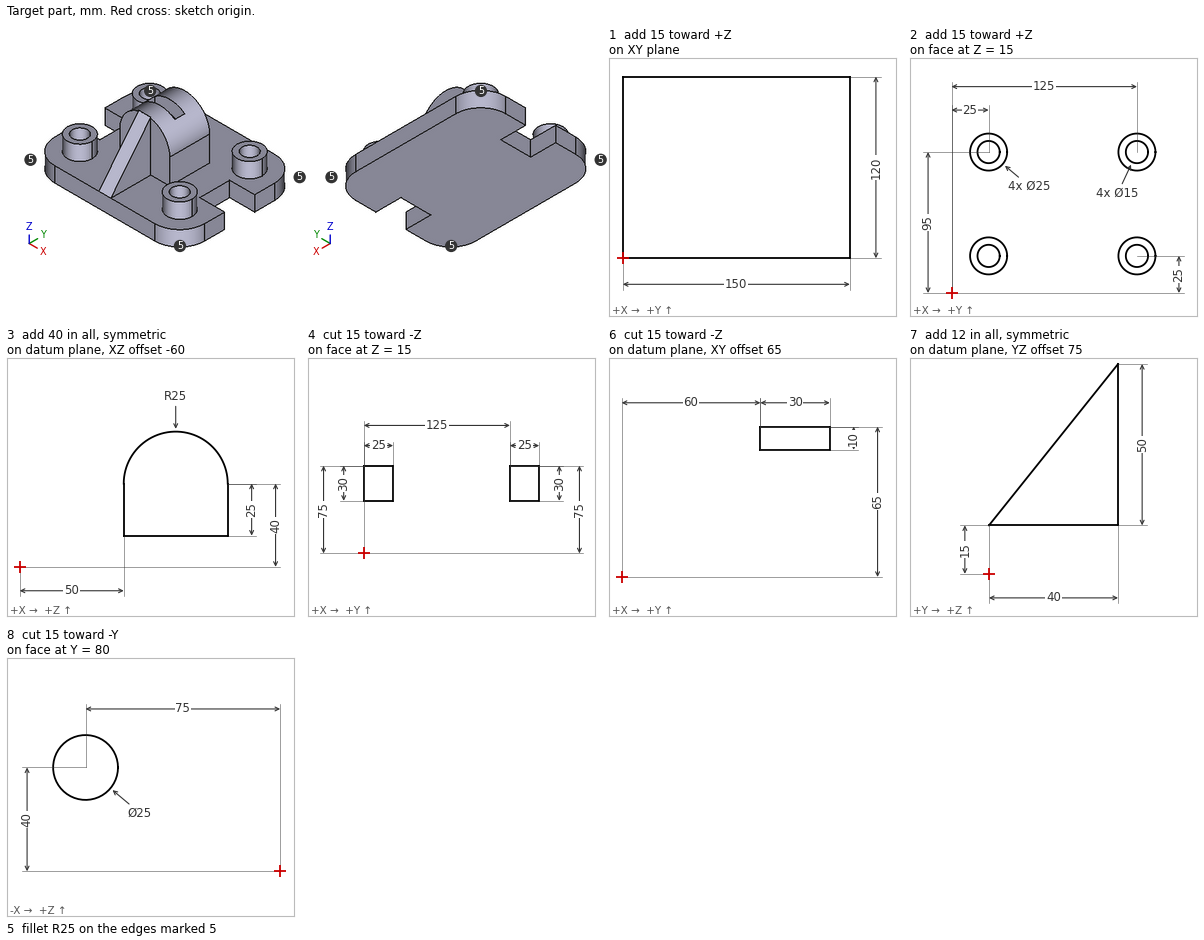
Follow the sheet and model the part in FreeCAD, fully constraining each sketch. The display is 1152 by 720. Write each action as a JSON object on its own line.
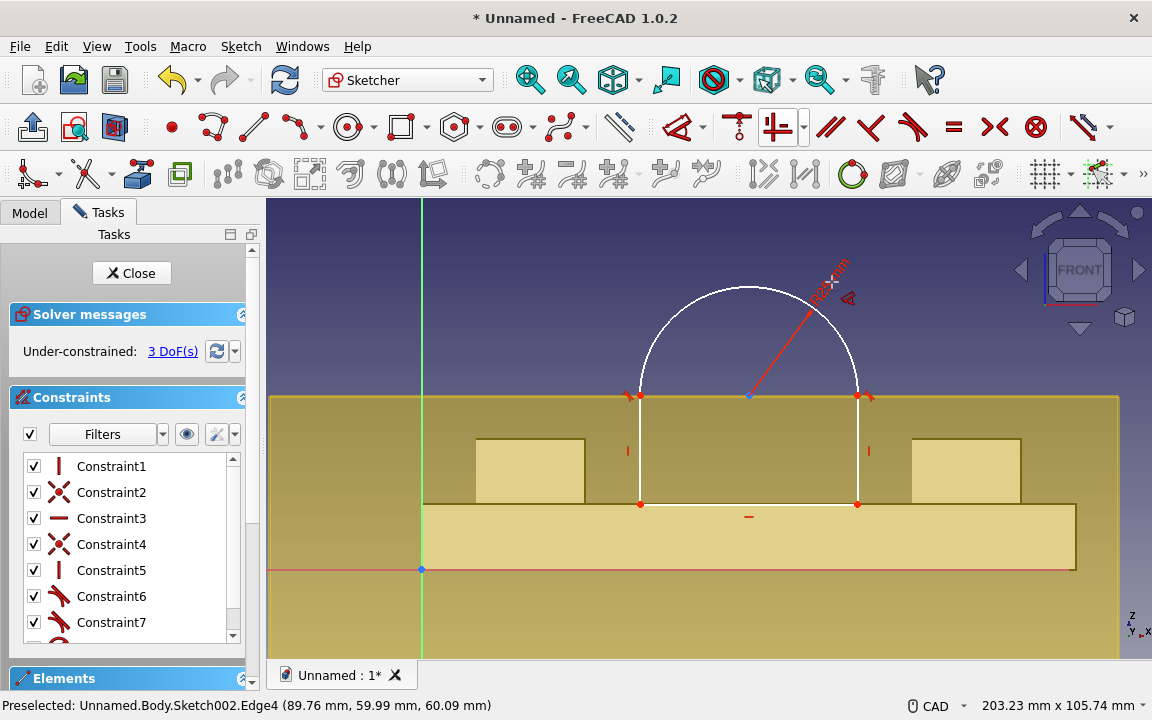
{"action": "left_click", "coordinate": [858, 429]}
{"action": "left_click", "coordinate": [892, 450]}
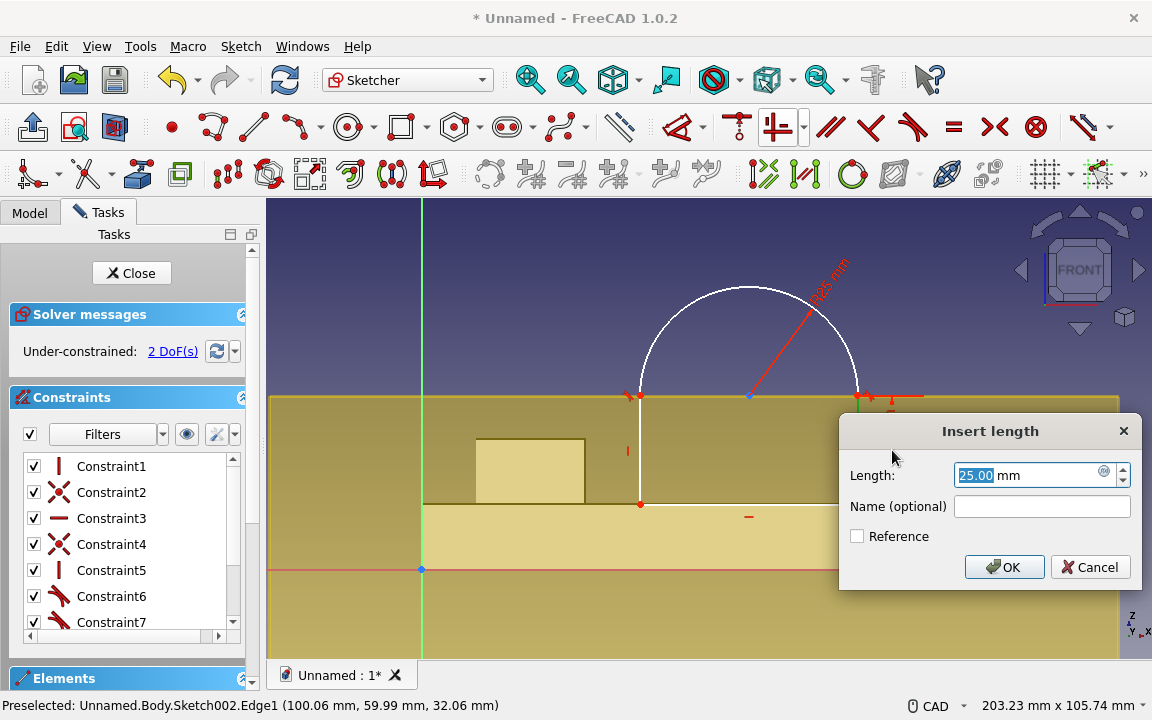
{"action": "type", "text": "25"}
{"action": "key", "text": "Return"}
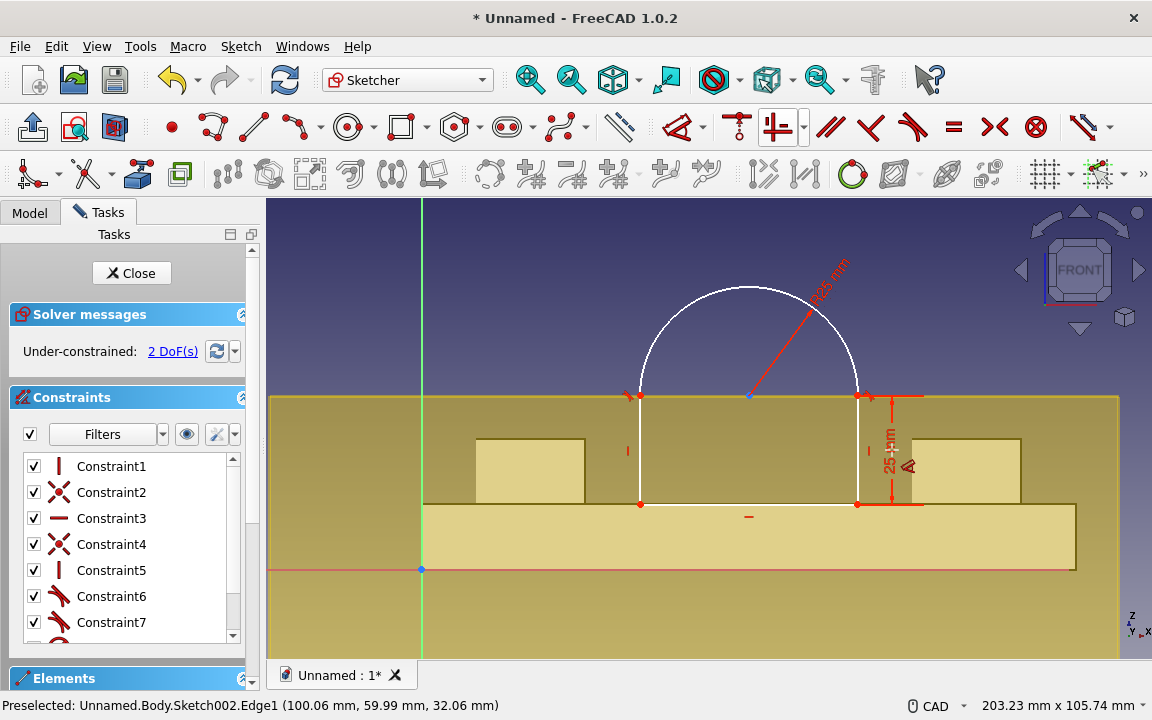
{"action": "left_click", "coordinate": [858, 396]}
{"action": "left_click", "coordinate": [892, 483]}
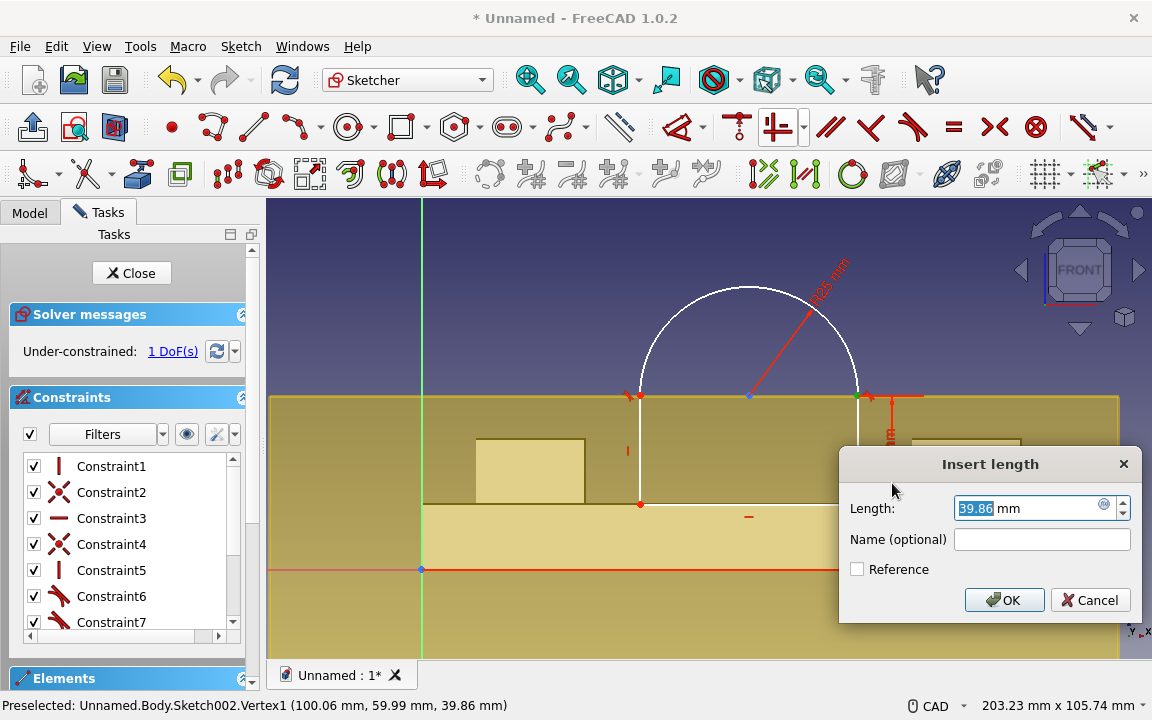
{"action": "type", "text": "40"}
{"action": "key", "text": "Return"}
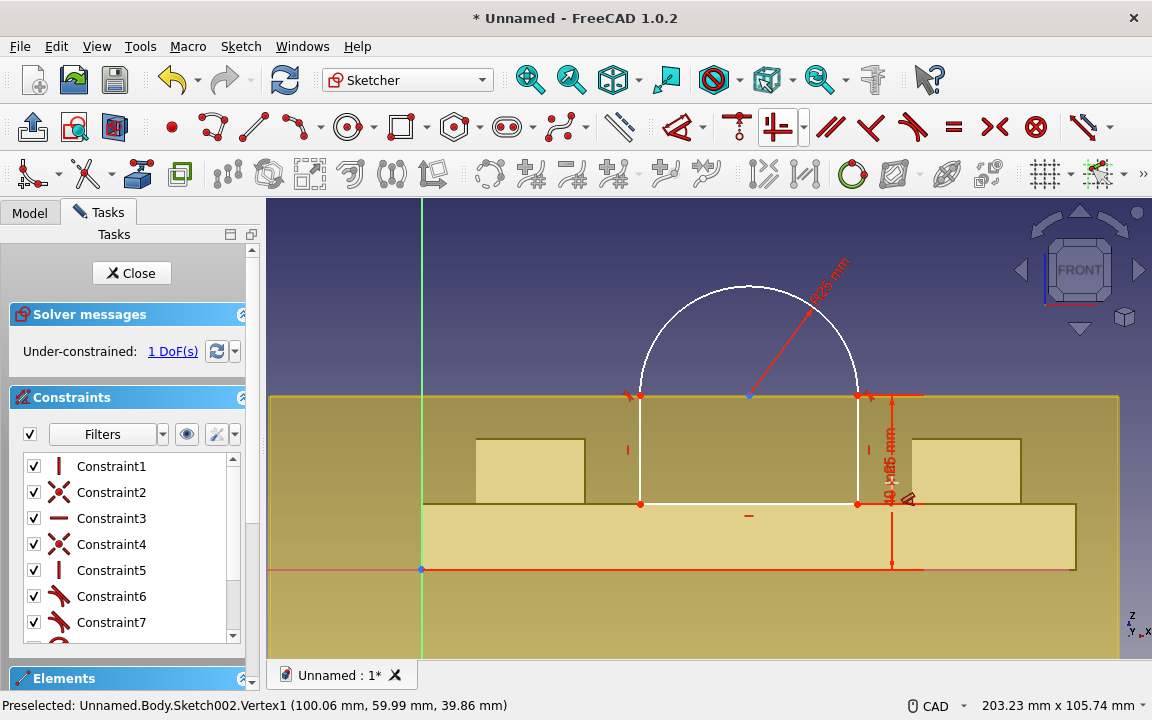
{"action": "left_click", "coordinate": [640, 504]}
{"action": "left_click", "coordinate": [531, 604]}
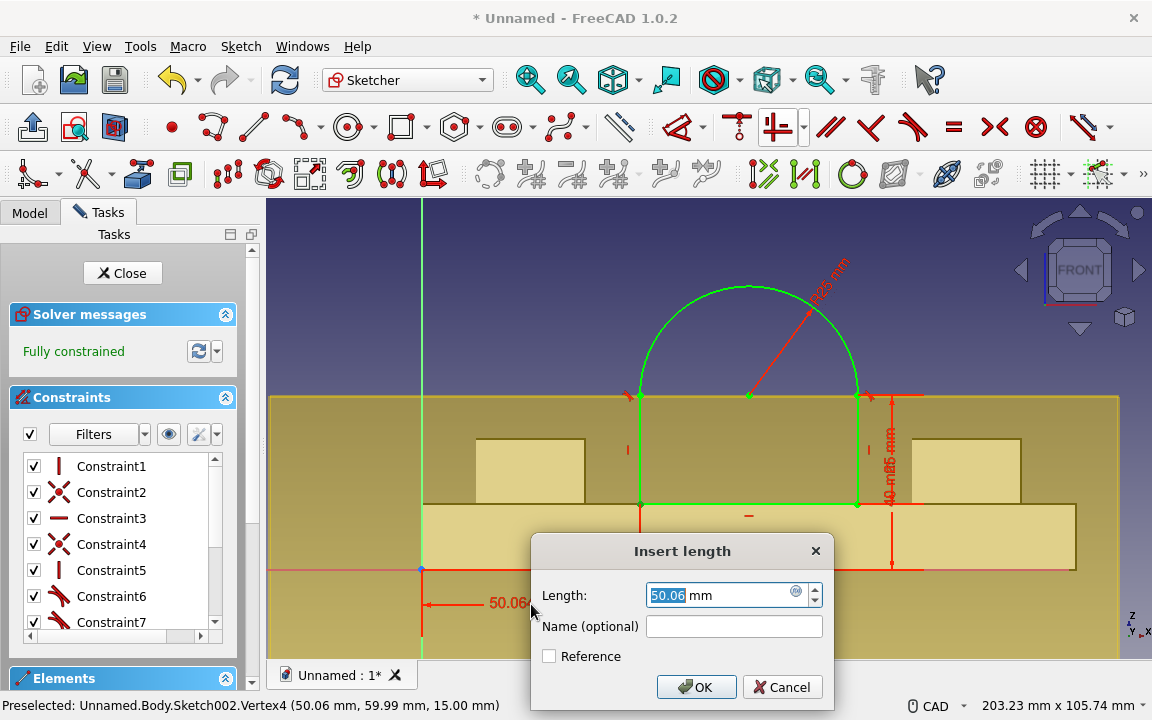
{"action": "type", "text": "50"}
{"action": "key", "text": "Return"}
{"action": "key", "text": "Escape"}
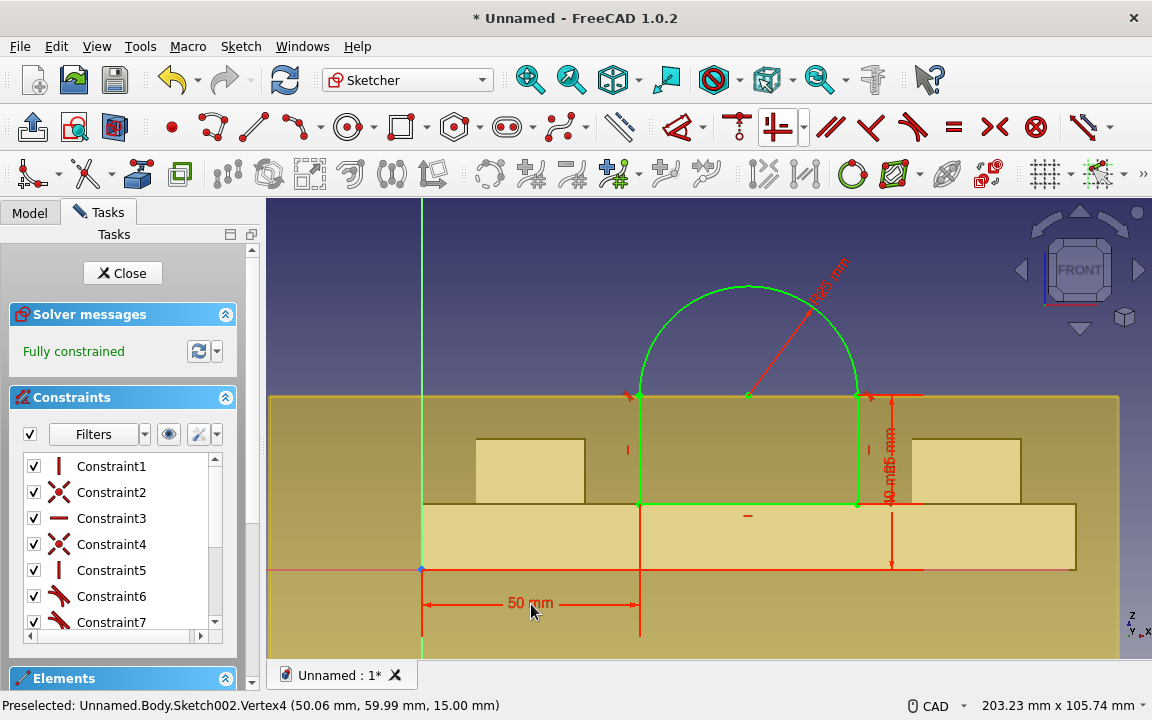
{"action": "left_click", "coordinate": [123, 273]}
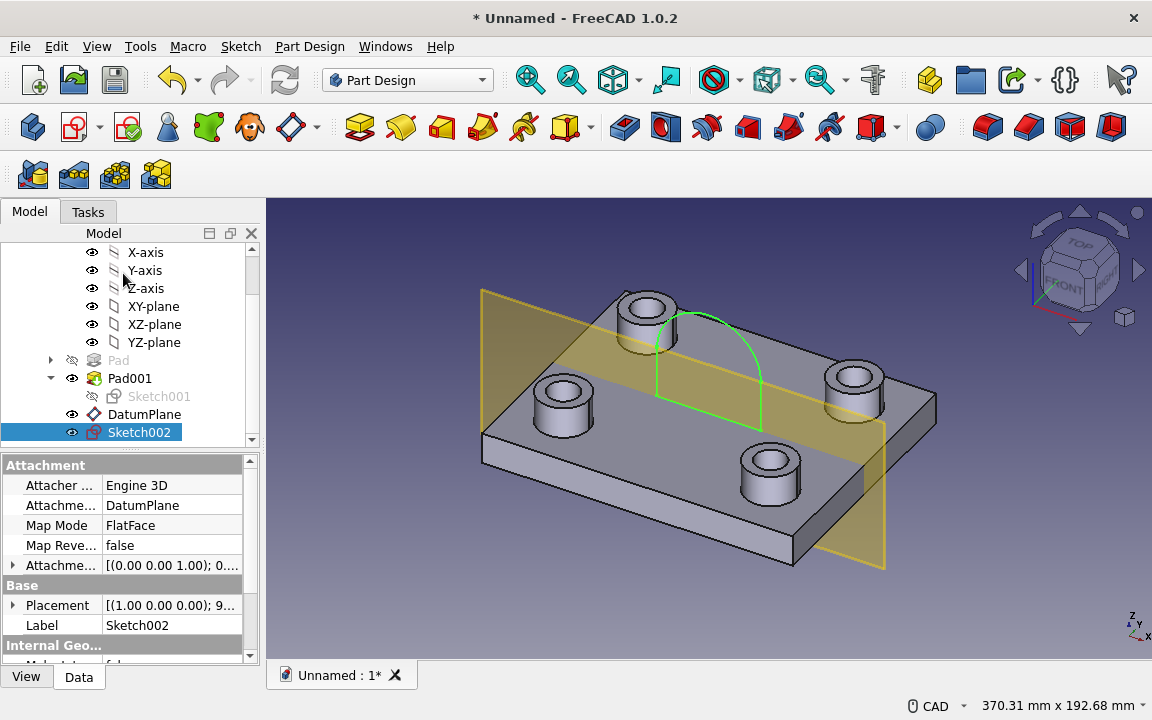
{"action": "left_click", "coordinate": [360, 128]}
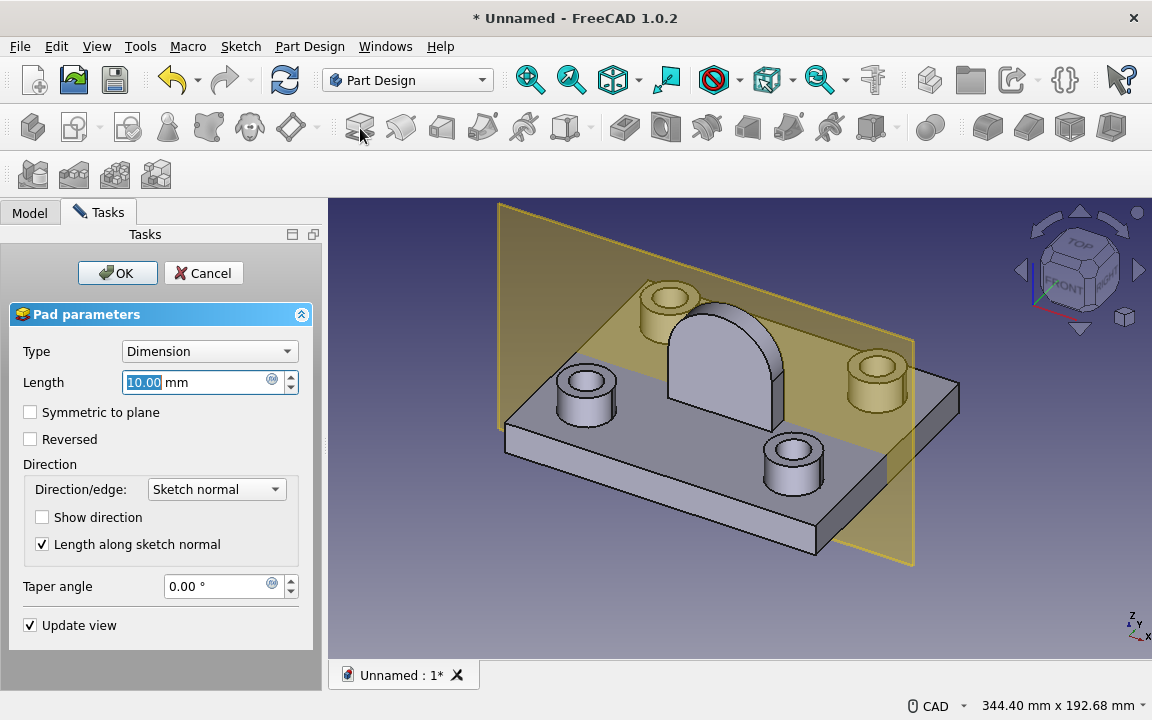
{"action": "type", "text": "40"}
{"action": "key", "text": "Tab"}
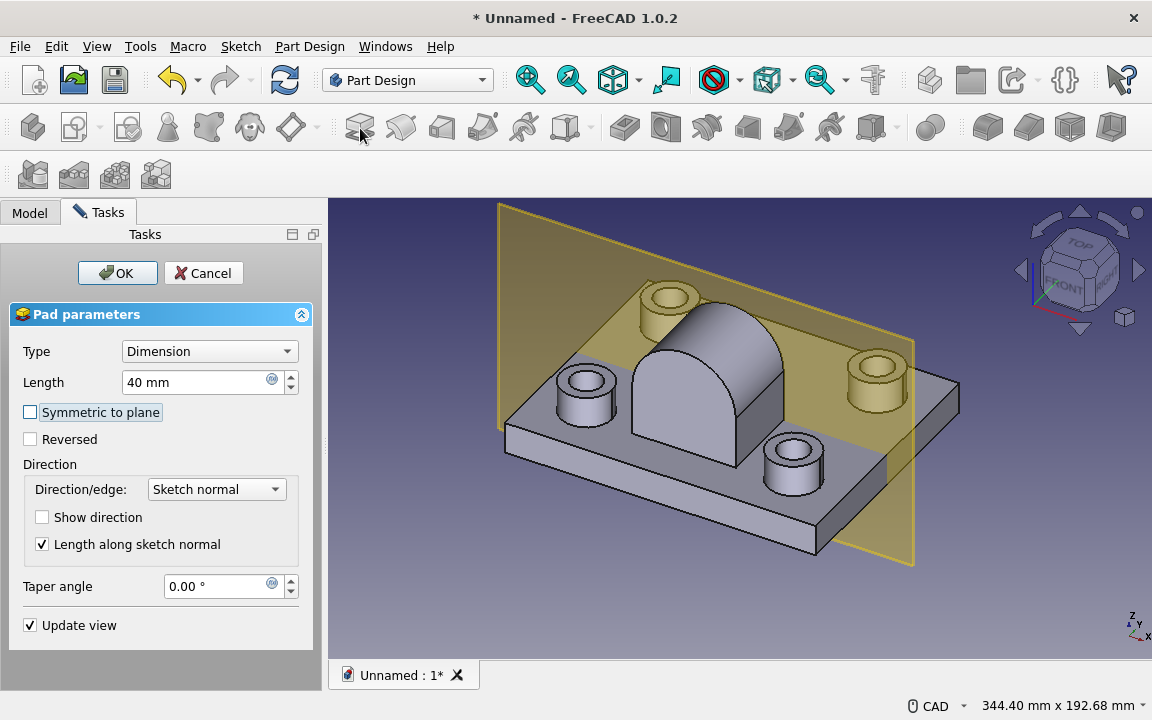
{"action": "left_click", "coordinate": [31, 412]}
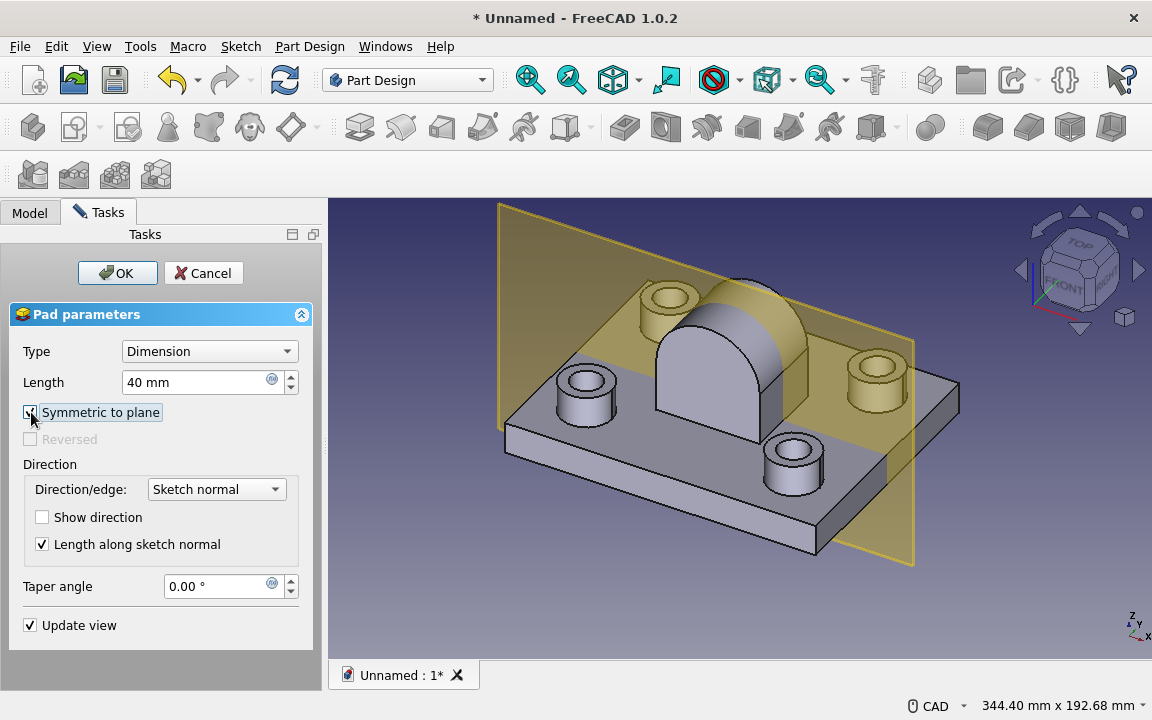
{"action": "left_click", "coordinate": [118, 273]}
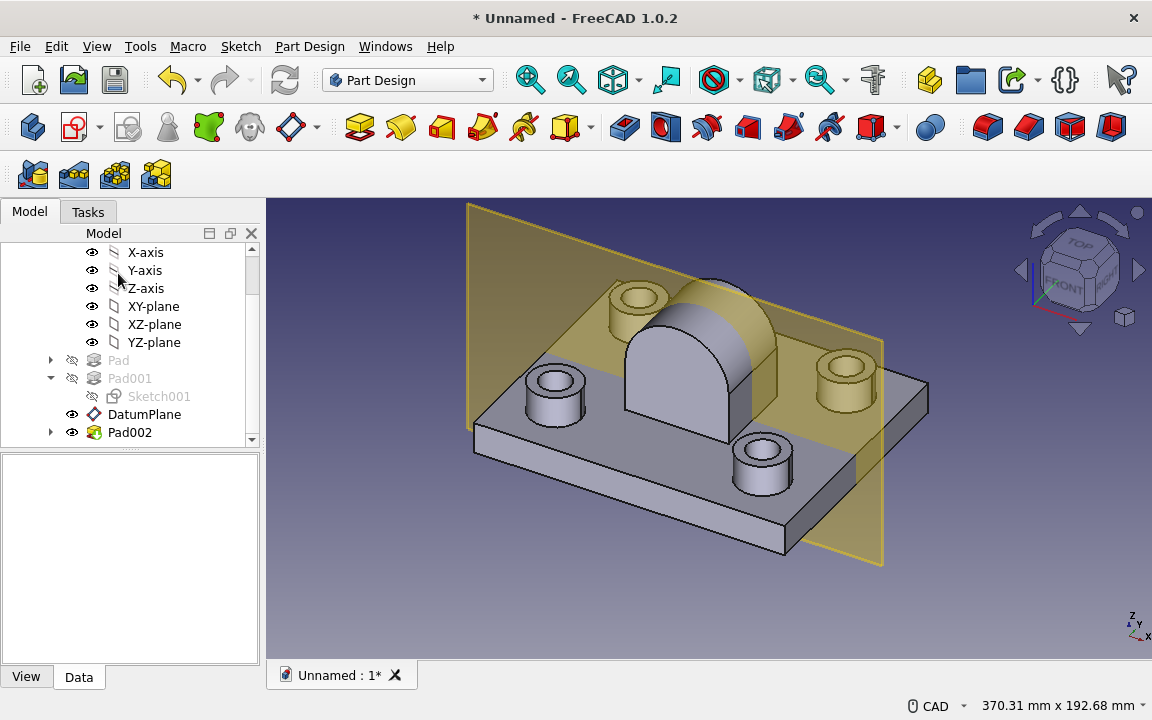
{"action": "left_click", "coordinate": [117, 414]}
{"action": "key", "text": "space"}